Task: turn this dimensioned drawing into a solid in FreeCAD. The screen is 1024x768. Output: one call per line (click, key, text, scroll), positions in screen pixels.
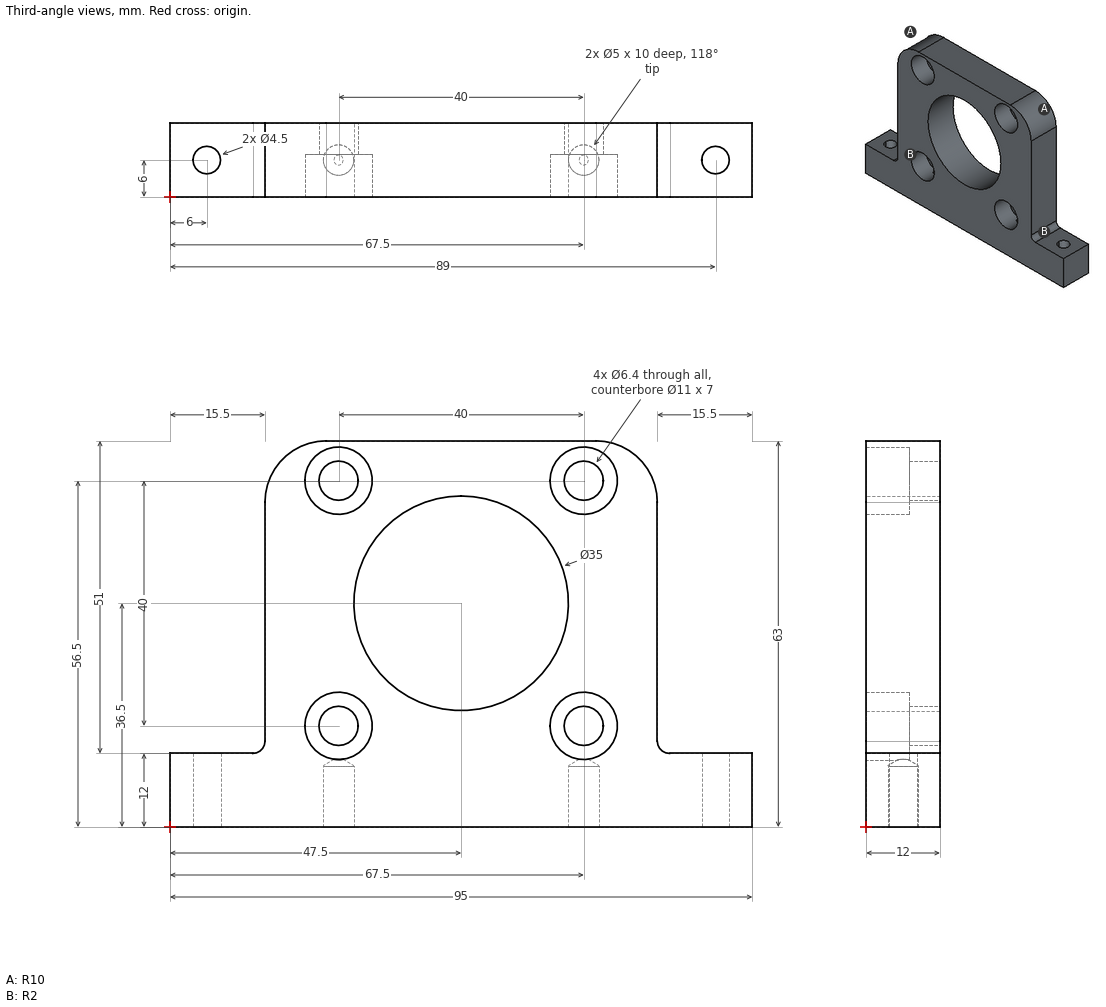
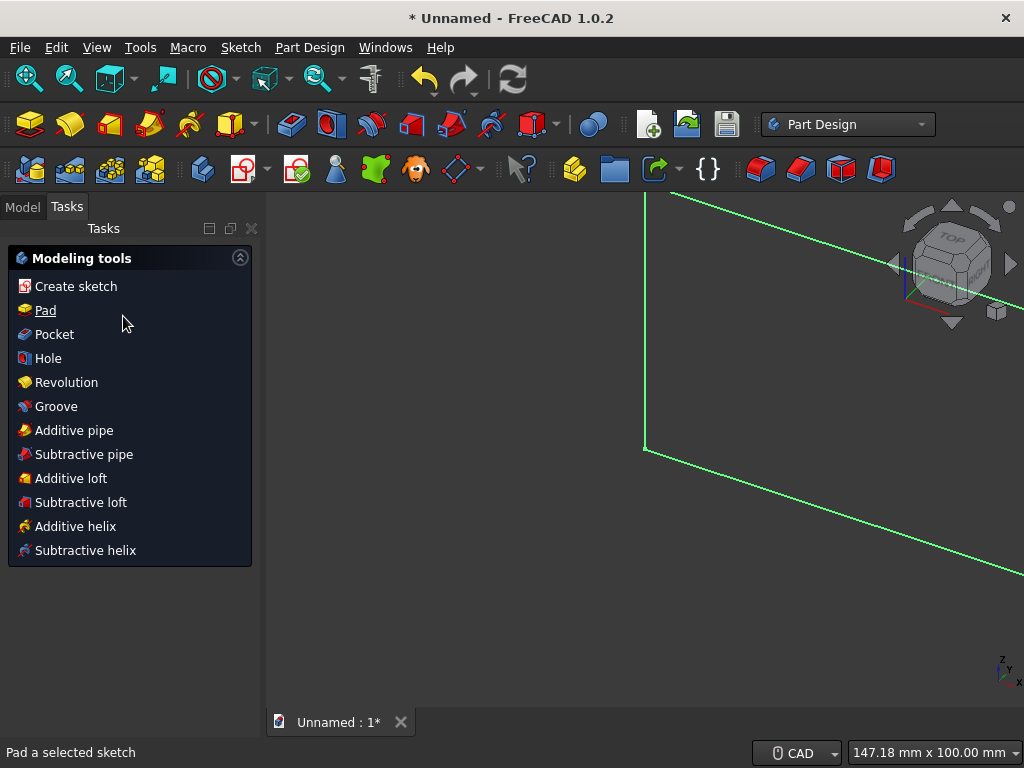
click(30, 124)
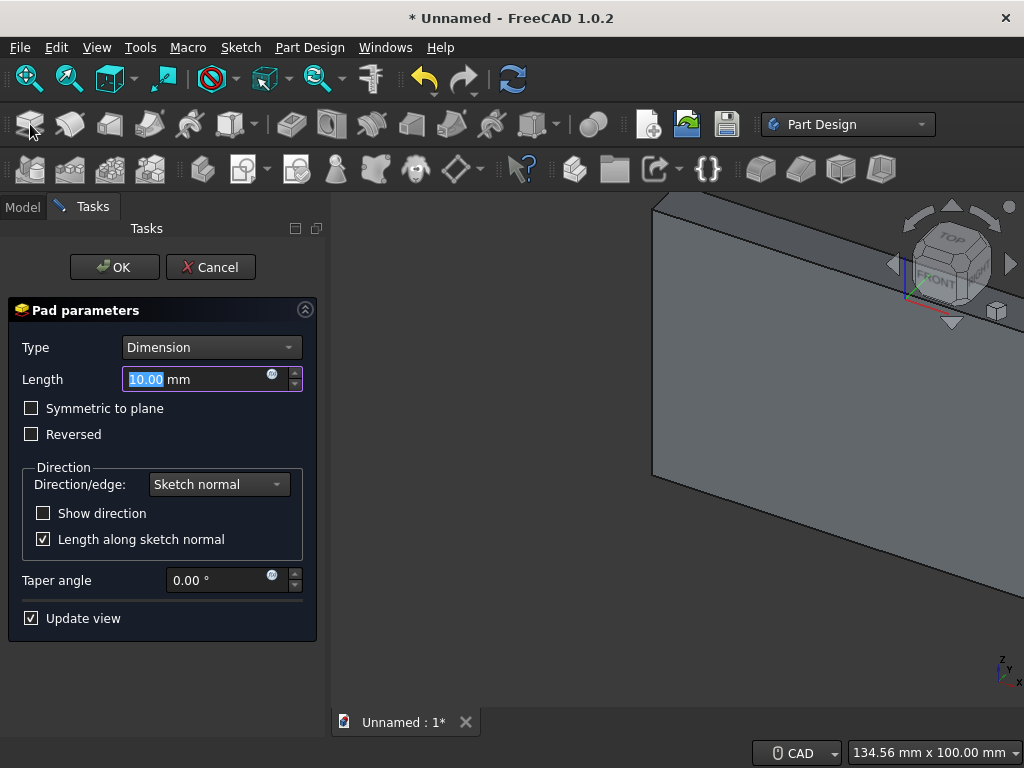
text(12)
key(Tab)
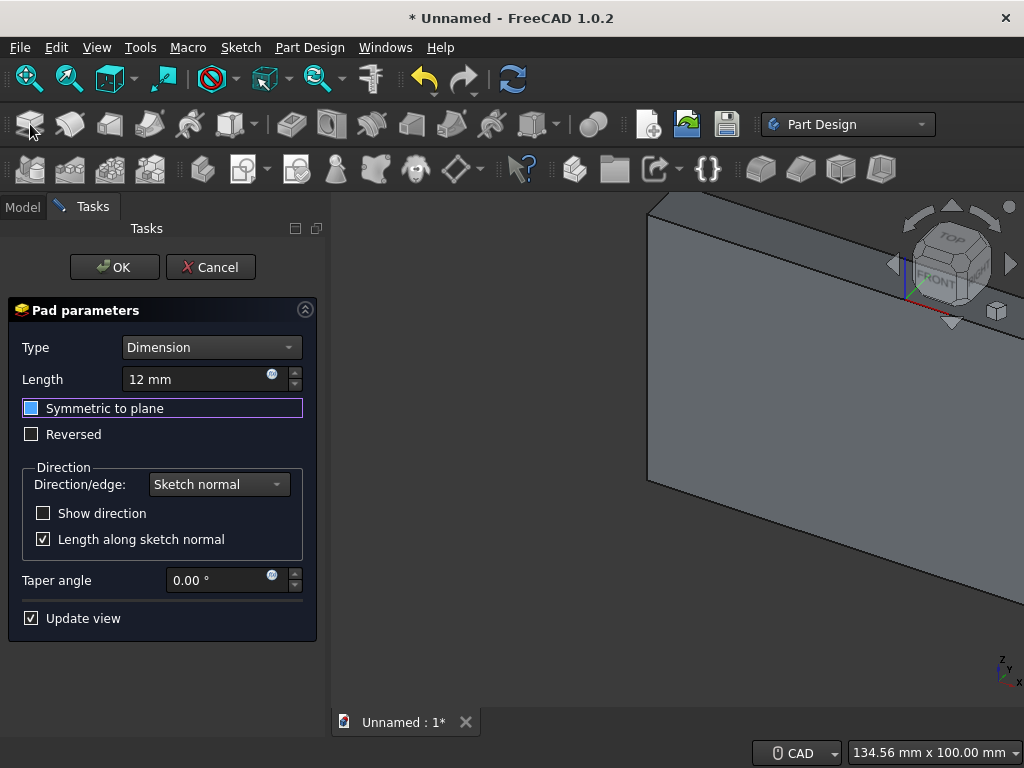
click(30, 434)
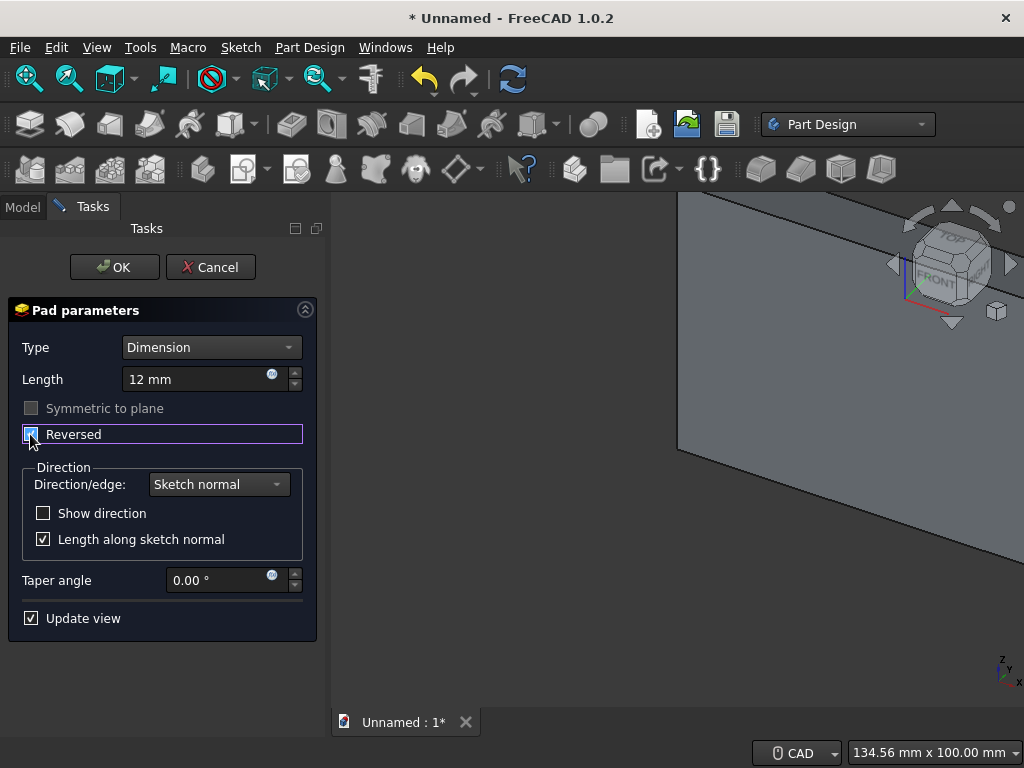
click(115, 267)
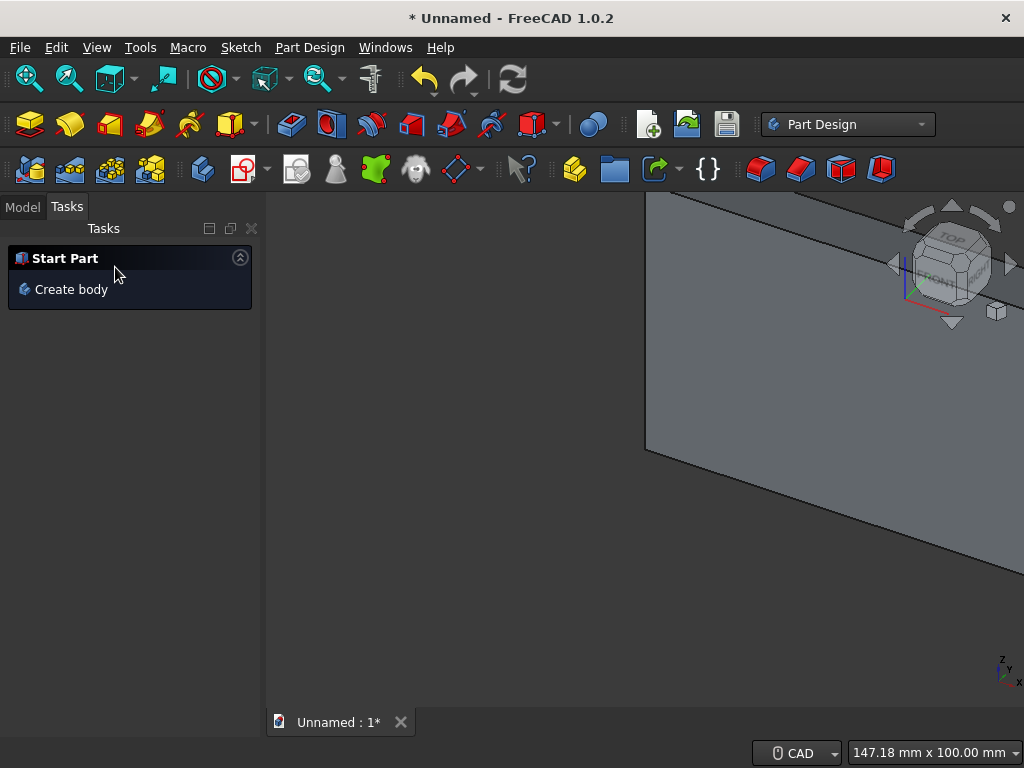
click(30, 80)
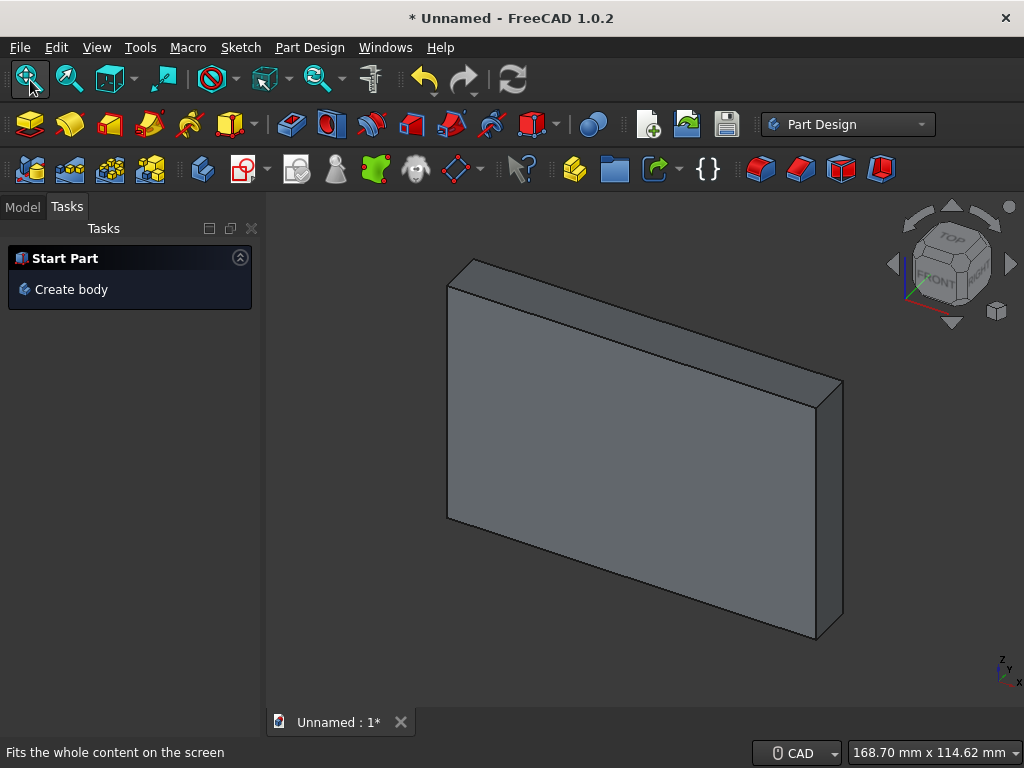
key(4)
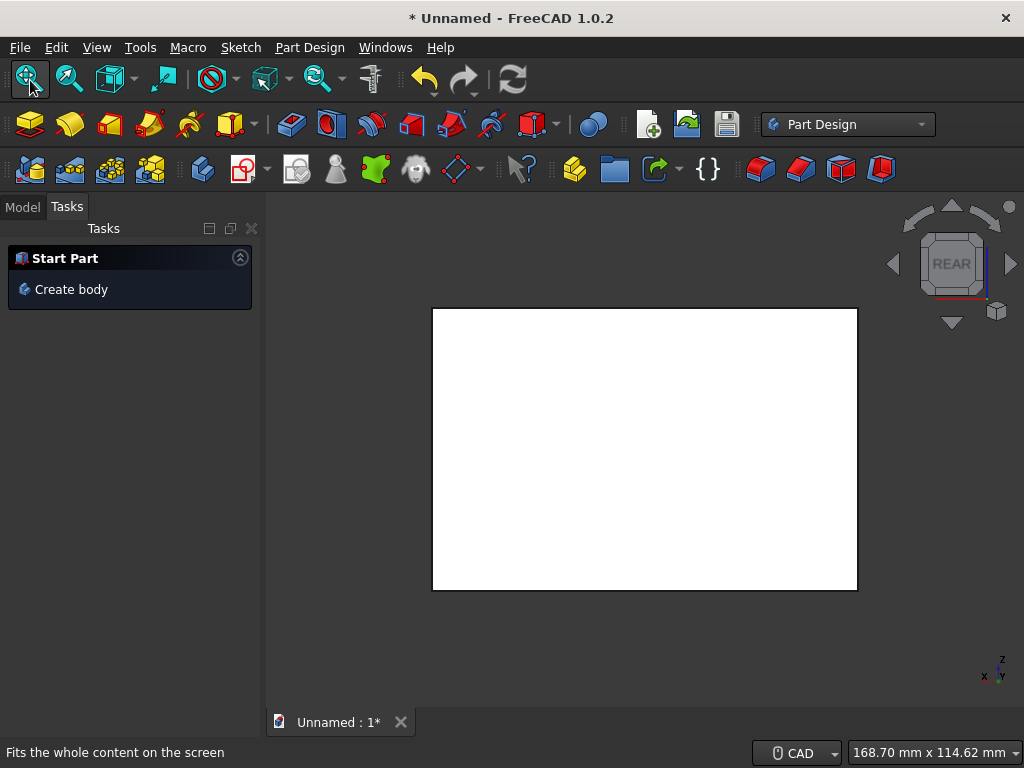
click(584, 449)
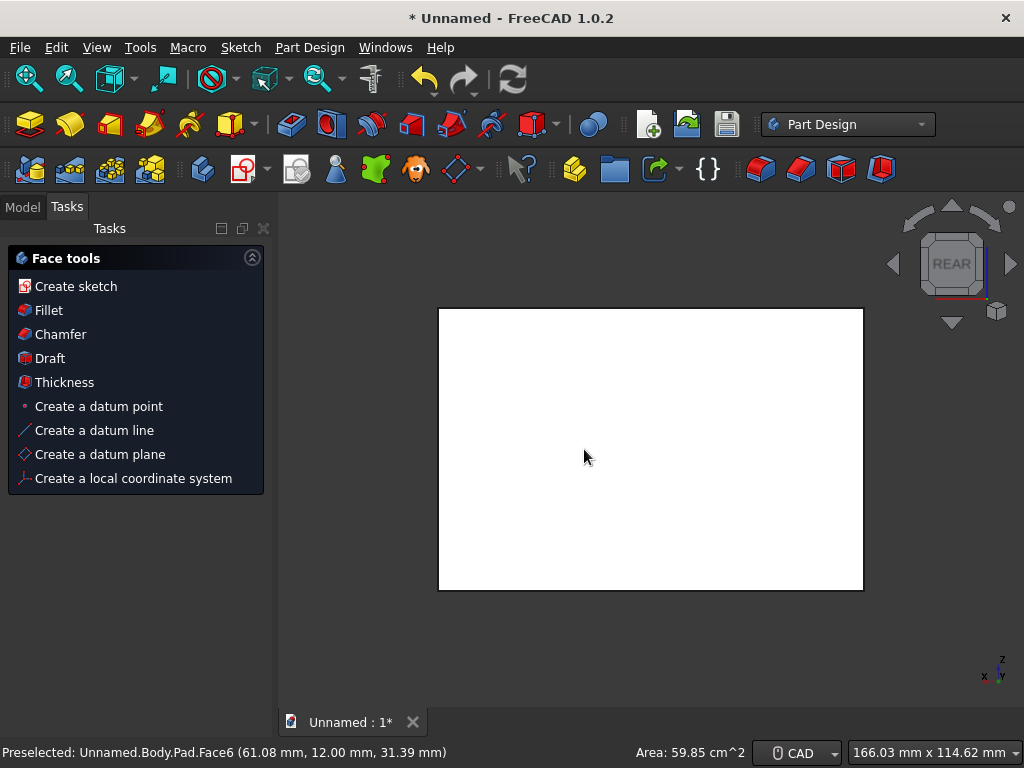
click(244, 170)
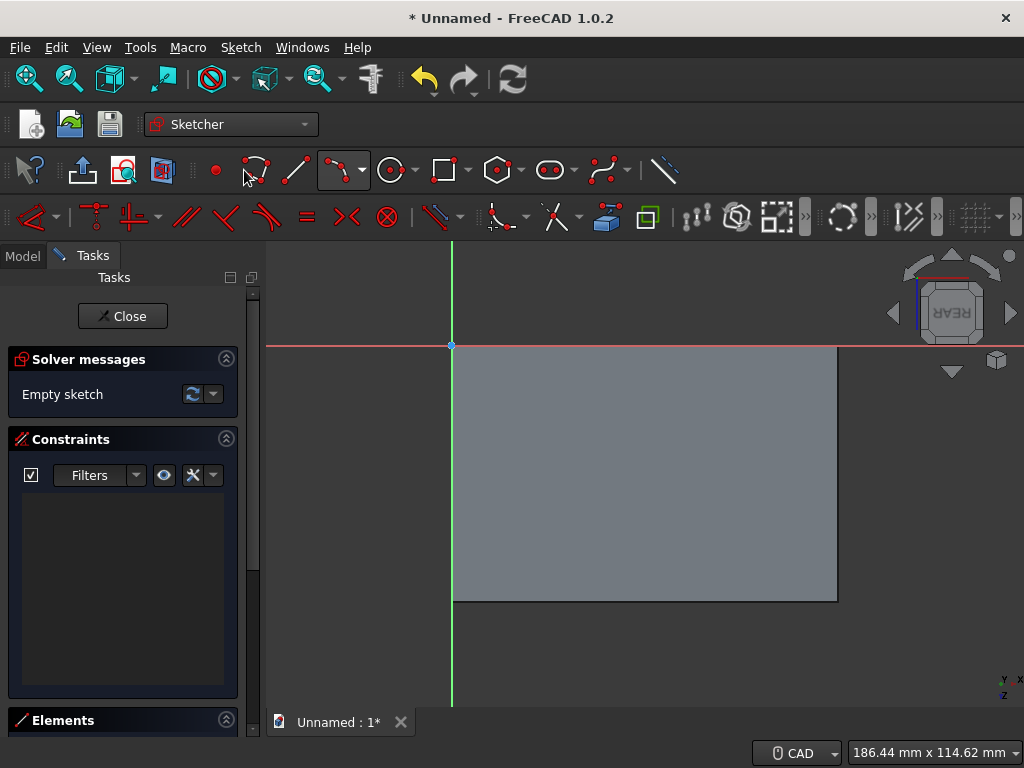
scroll(294, 474, down, 1)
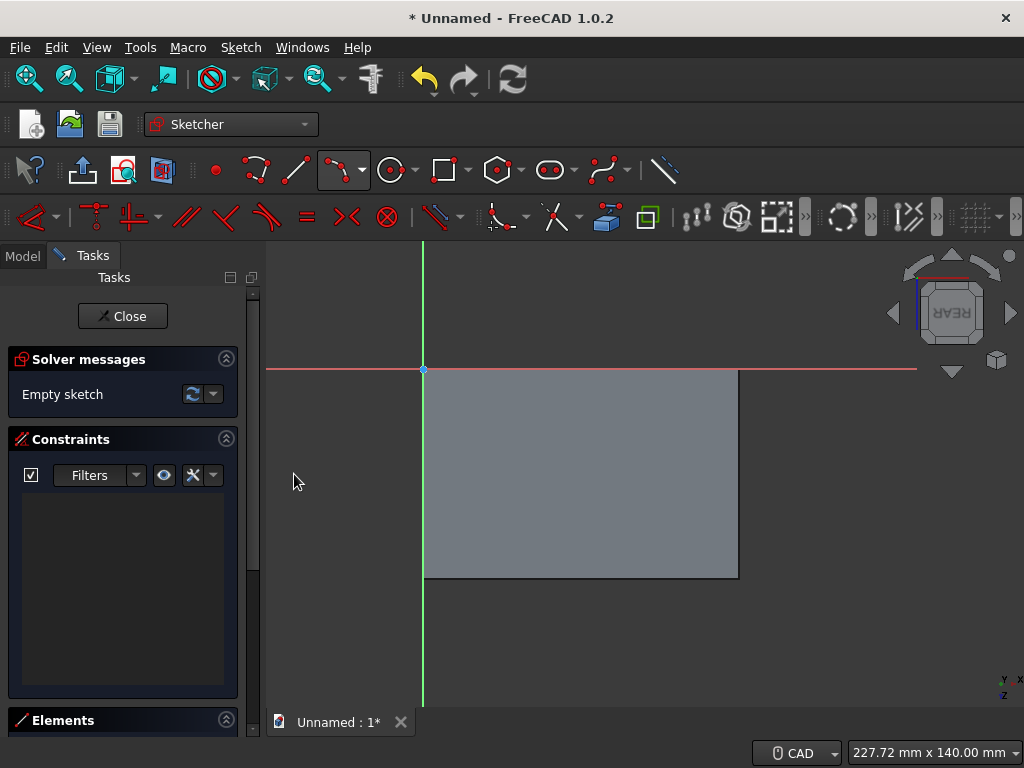
click(444, 170)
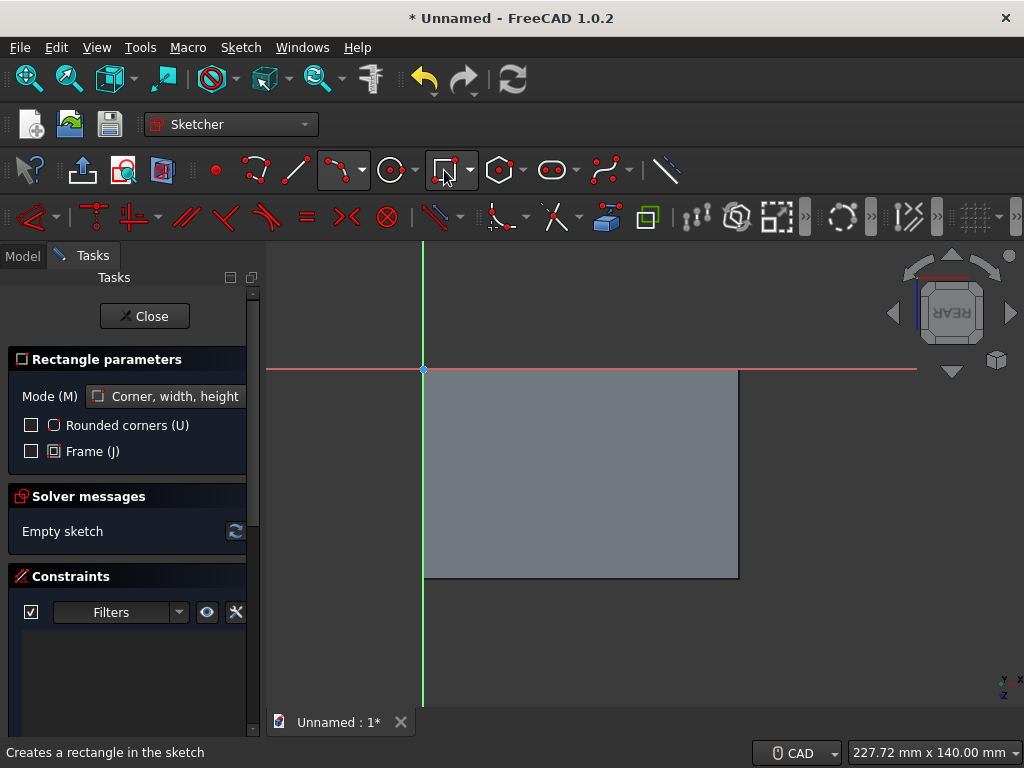
click(423, 409)
click(475, 579)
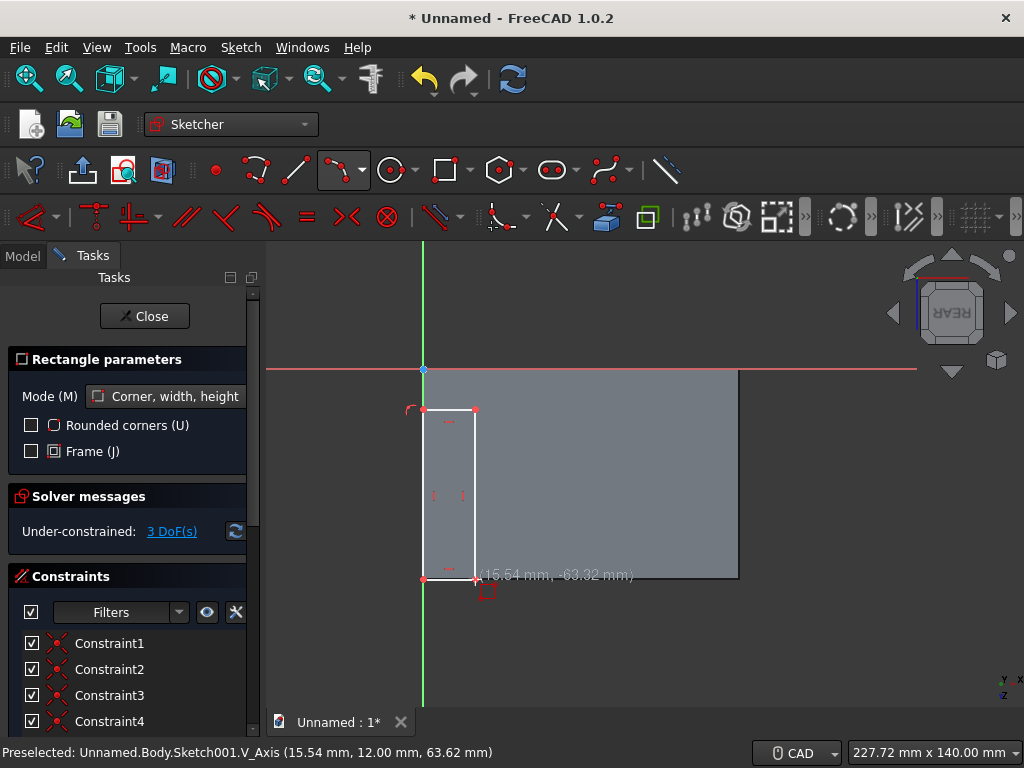
click(688, 409)
click(739, 579)
key(Escape)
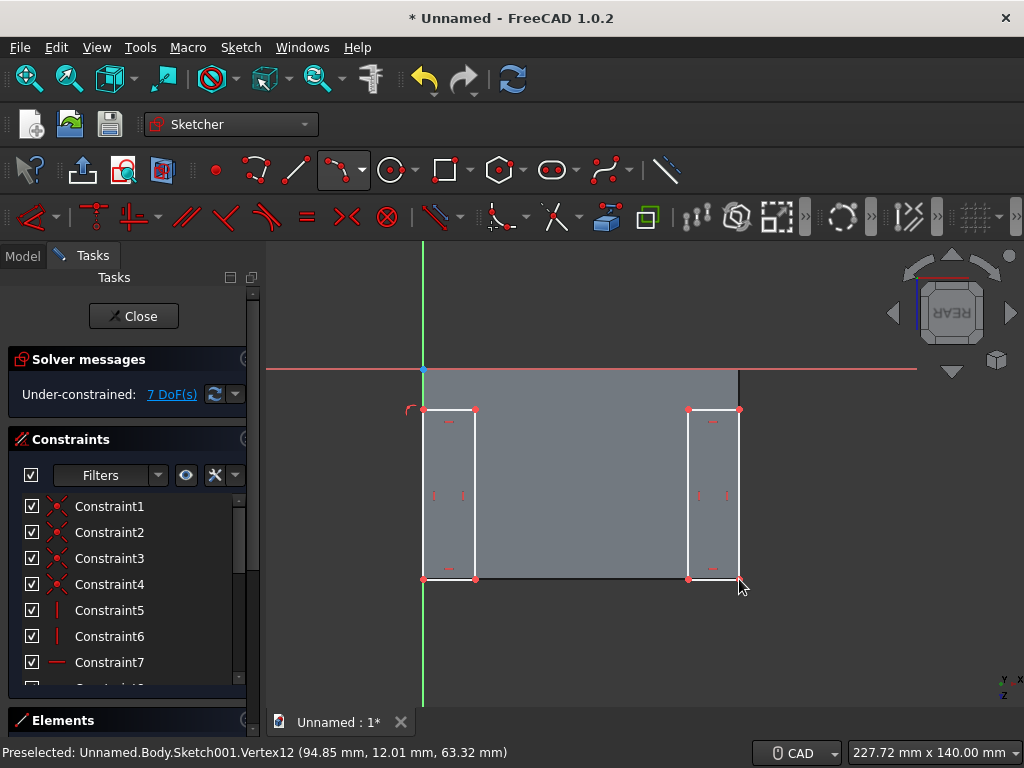
click(32, 218)